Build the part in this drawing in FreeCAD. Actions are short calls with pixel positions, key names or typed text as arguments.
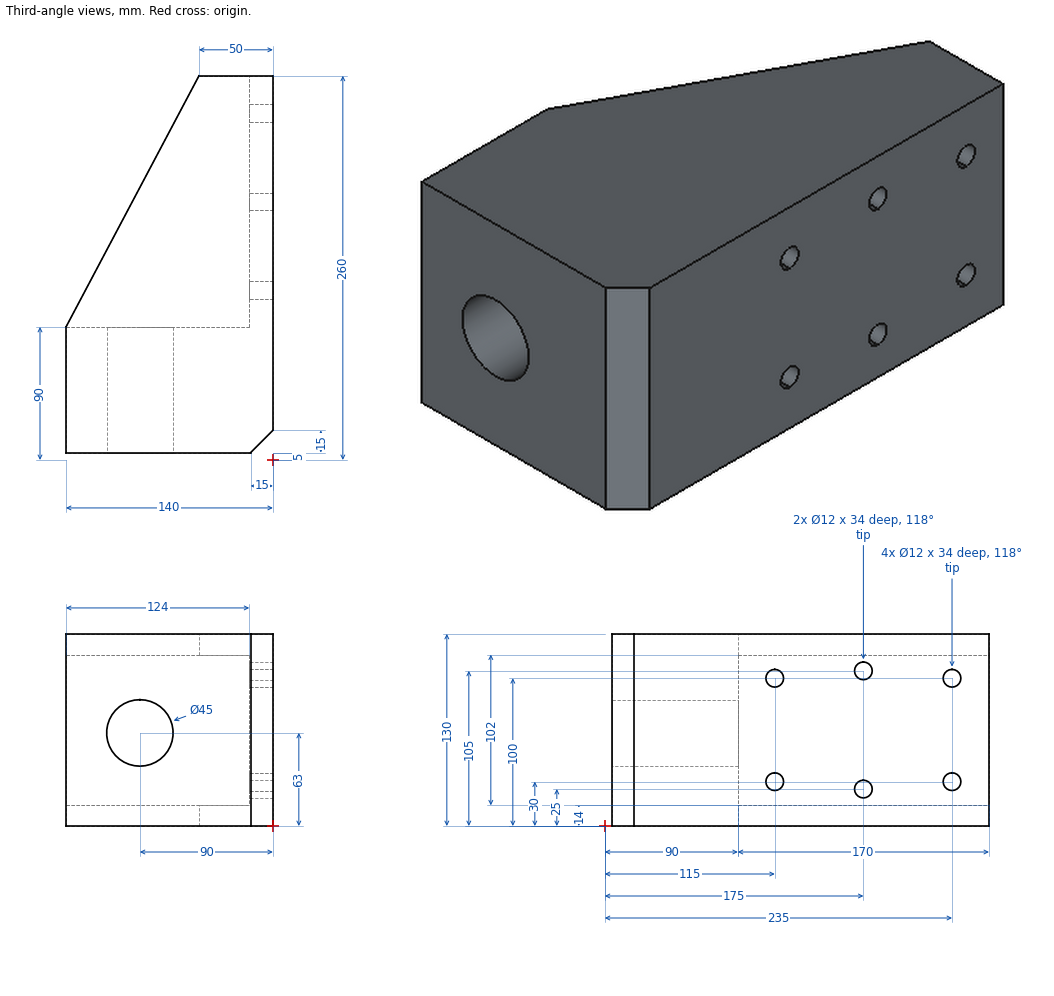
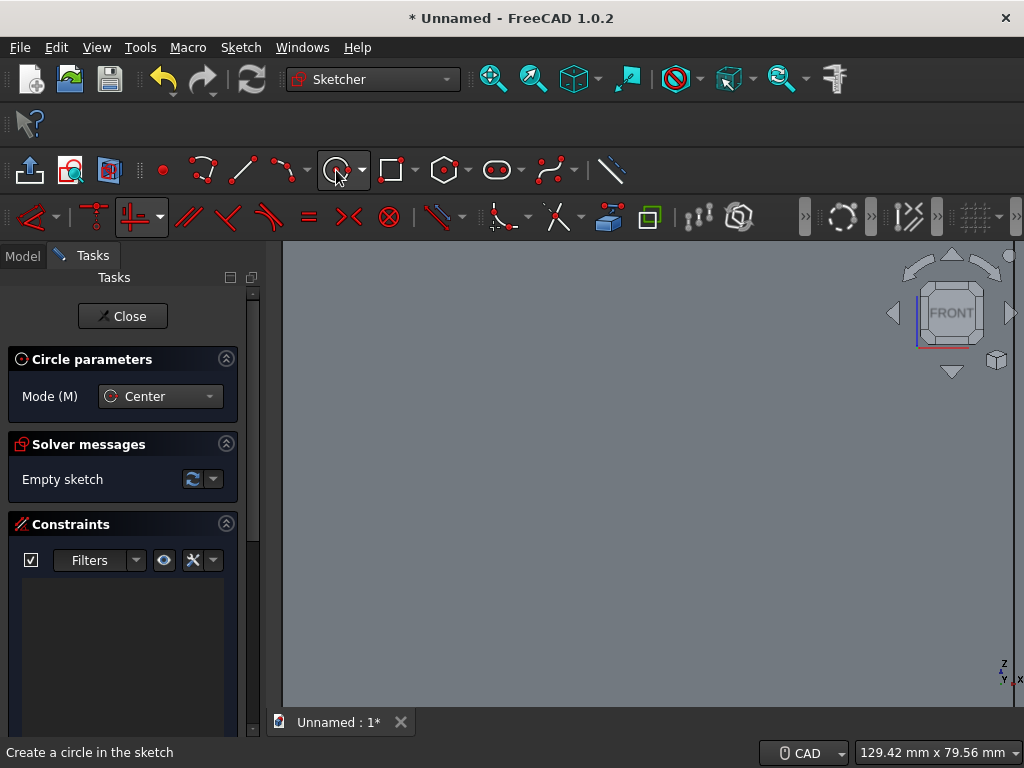
click(575, 472)
move(668, 379)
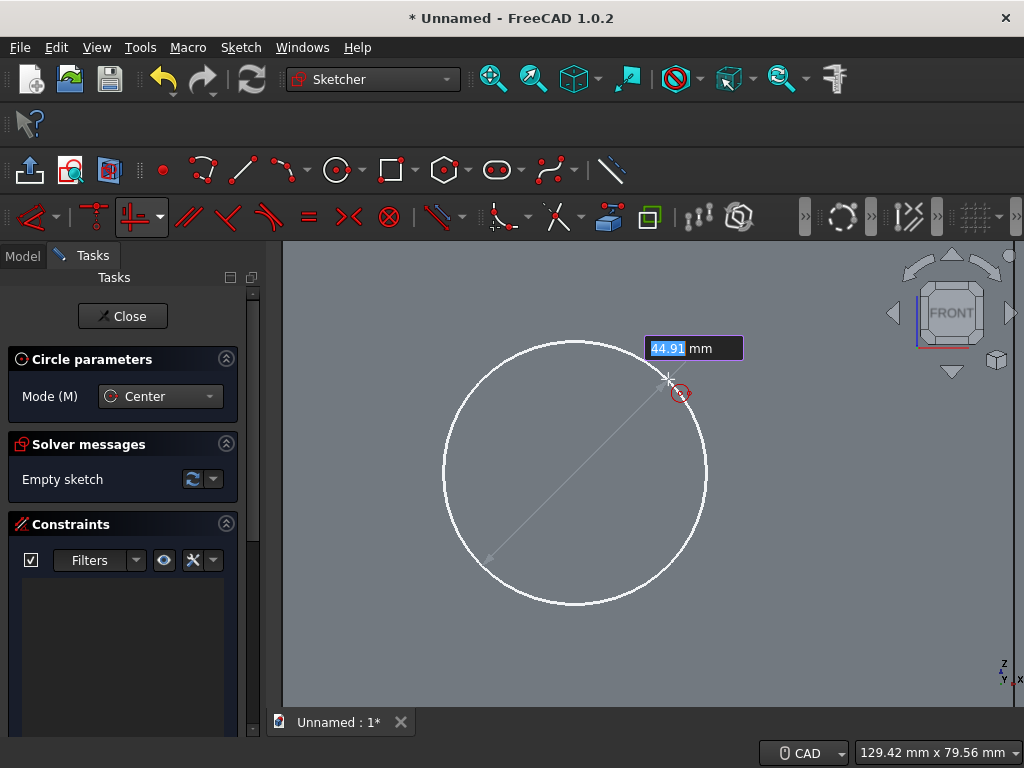
text(45)
key(Return)
key(Escape)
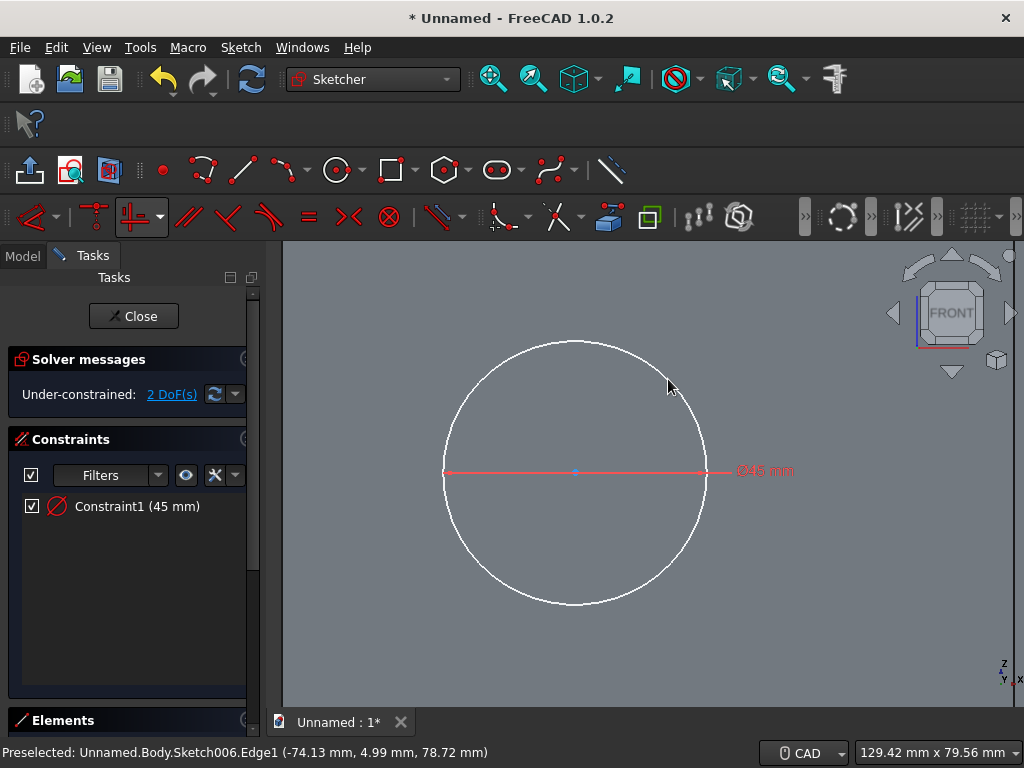
click(32, 218)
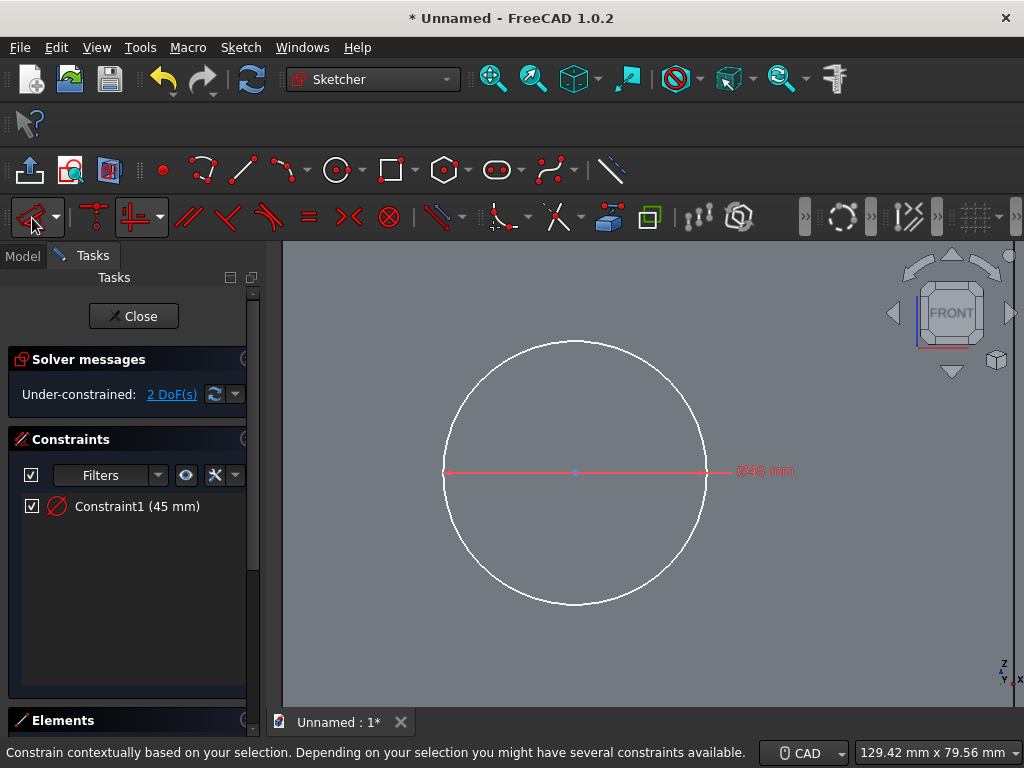
click(575, 473)
click(717, 439)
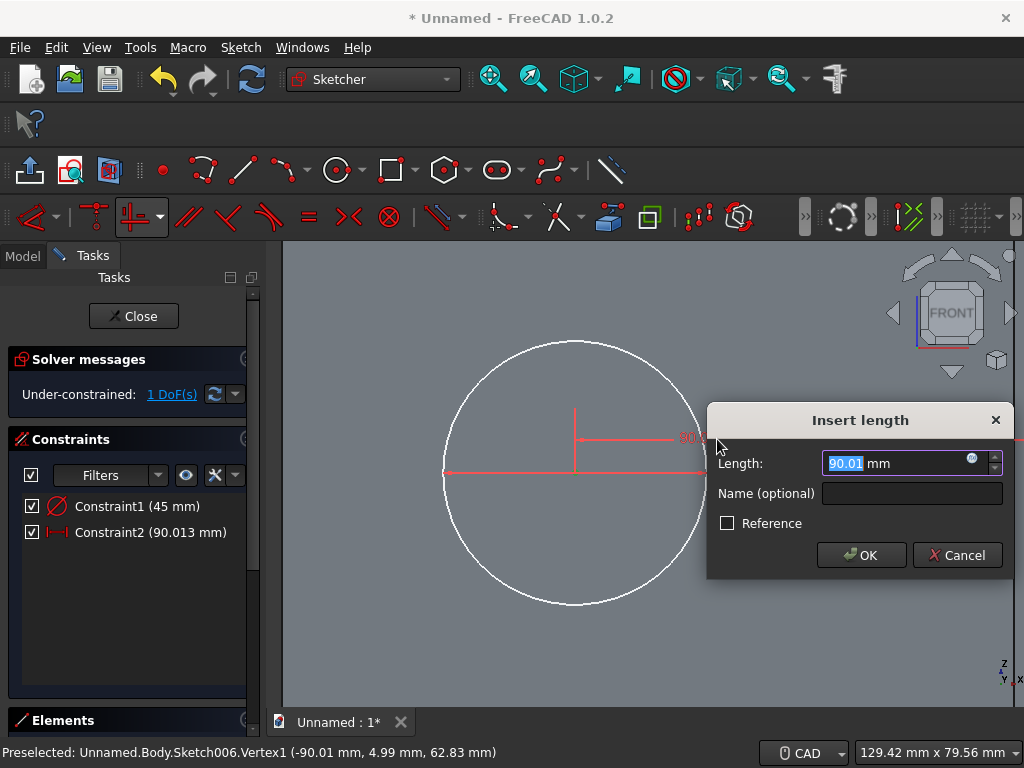
text(90)
key(Return)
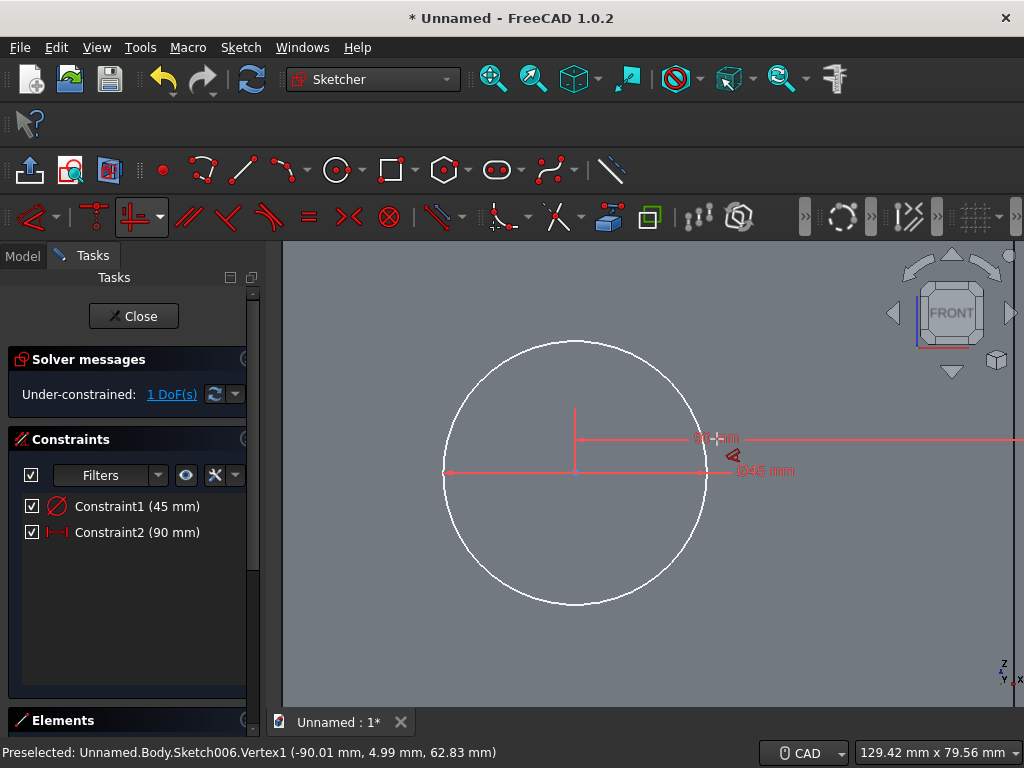
click(575, 473)
click(541, 576)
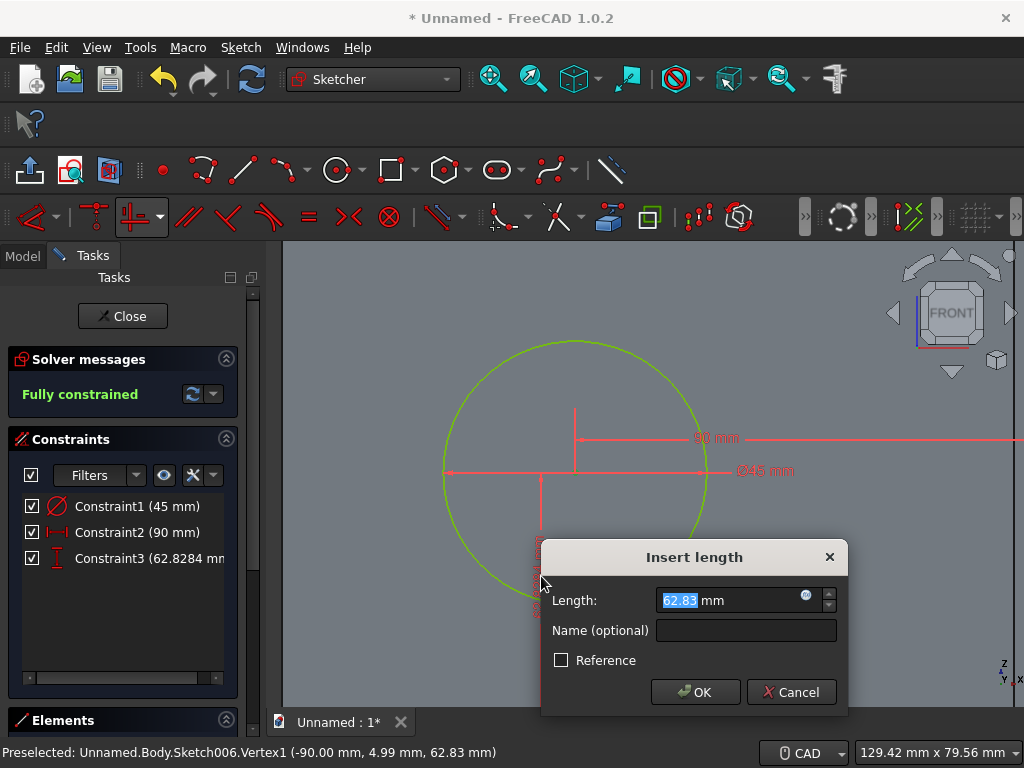
text(63)
key(Return)
key(Escape)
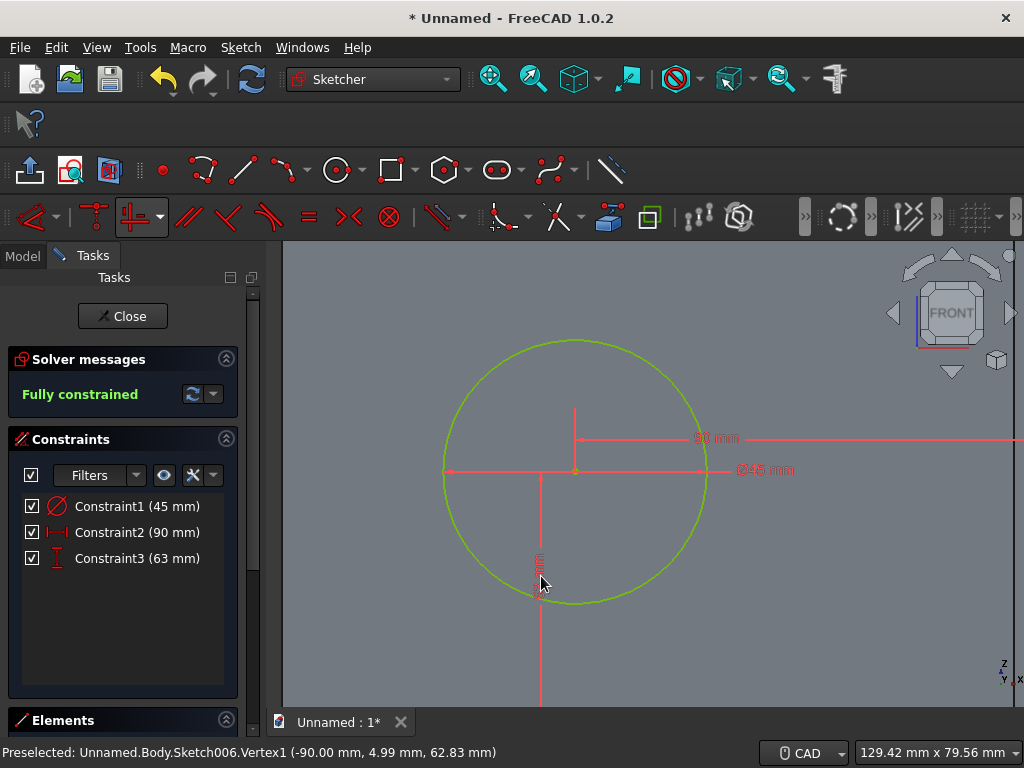
click(123, 316)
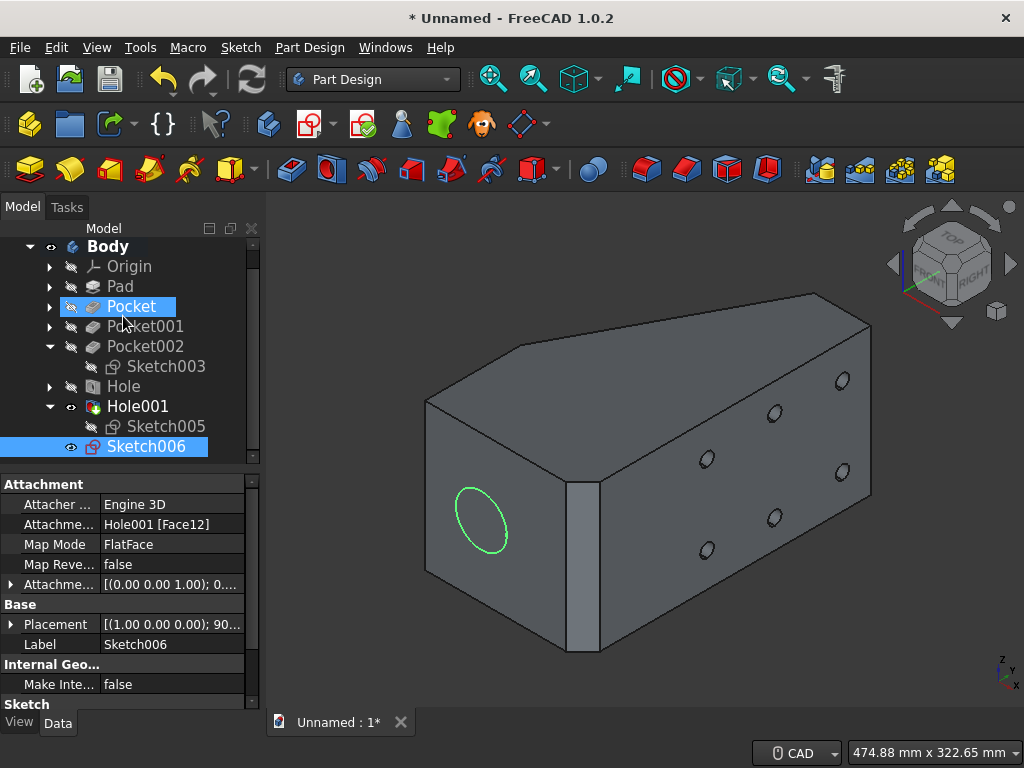
click(292, 170)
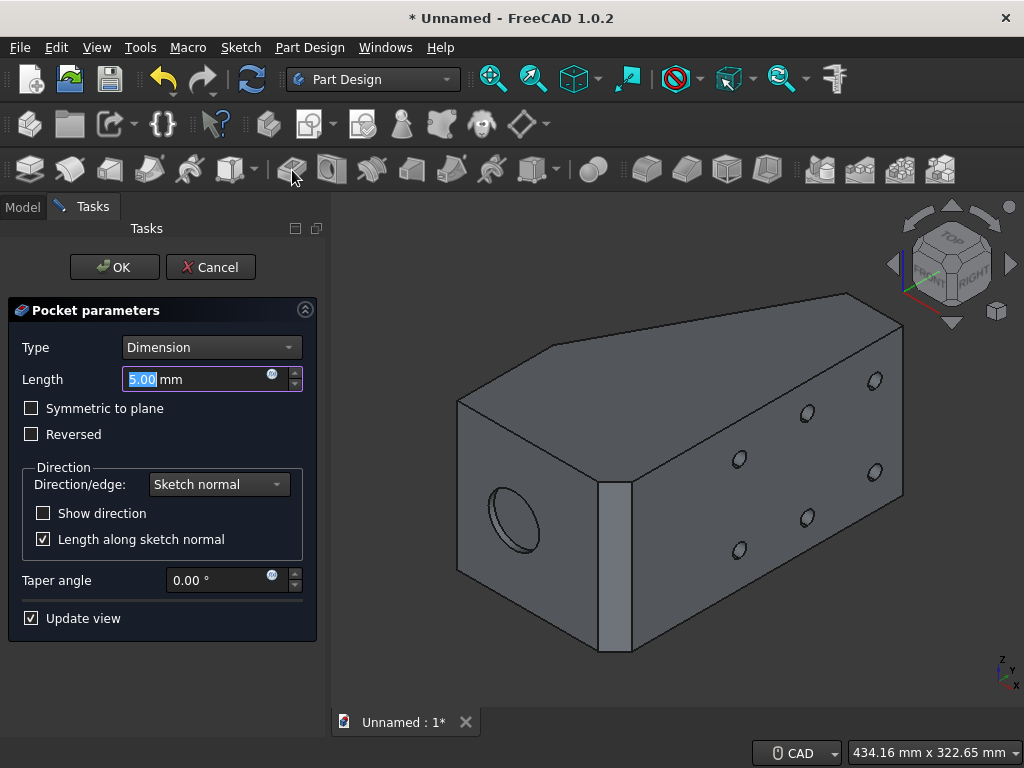
click(212, 348)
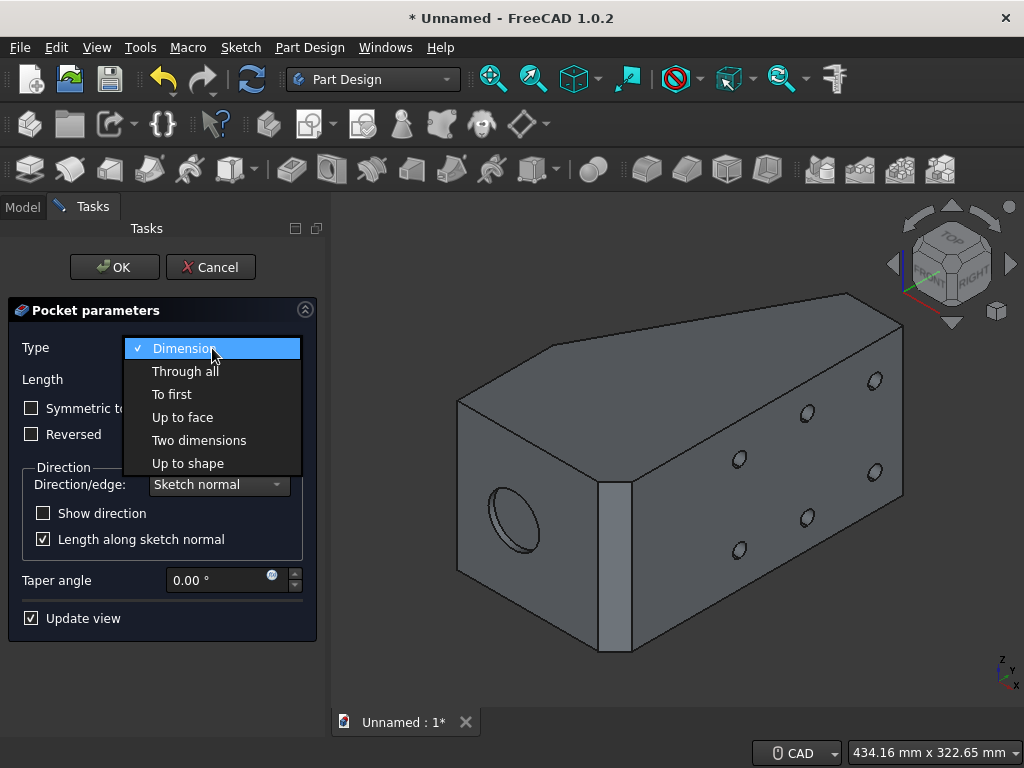
click(212, 394)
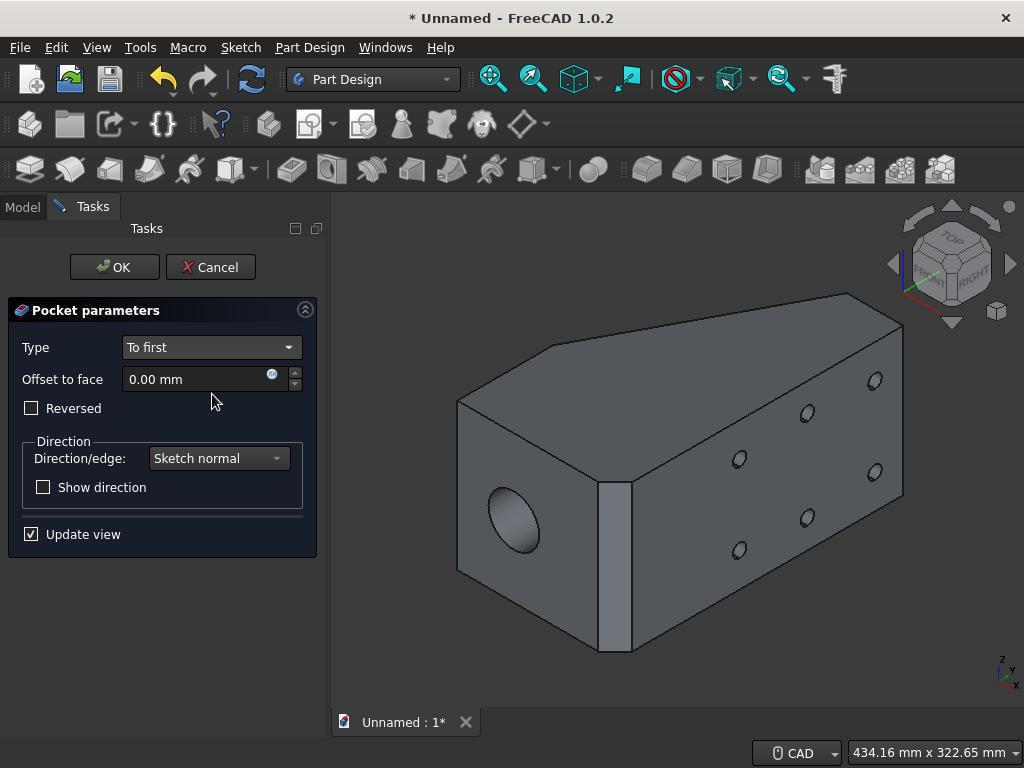
click(115, 267)